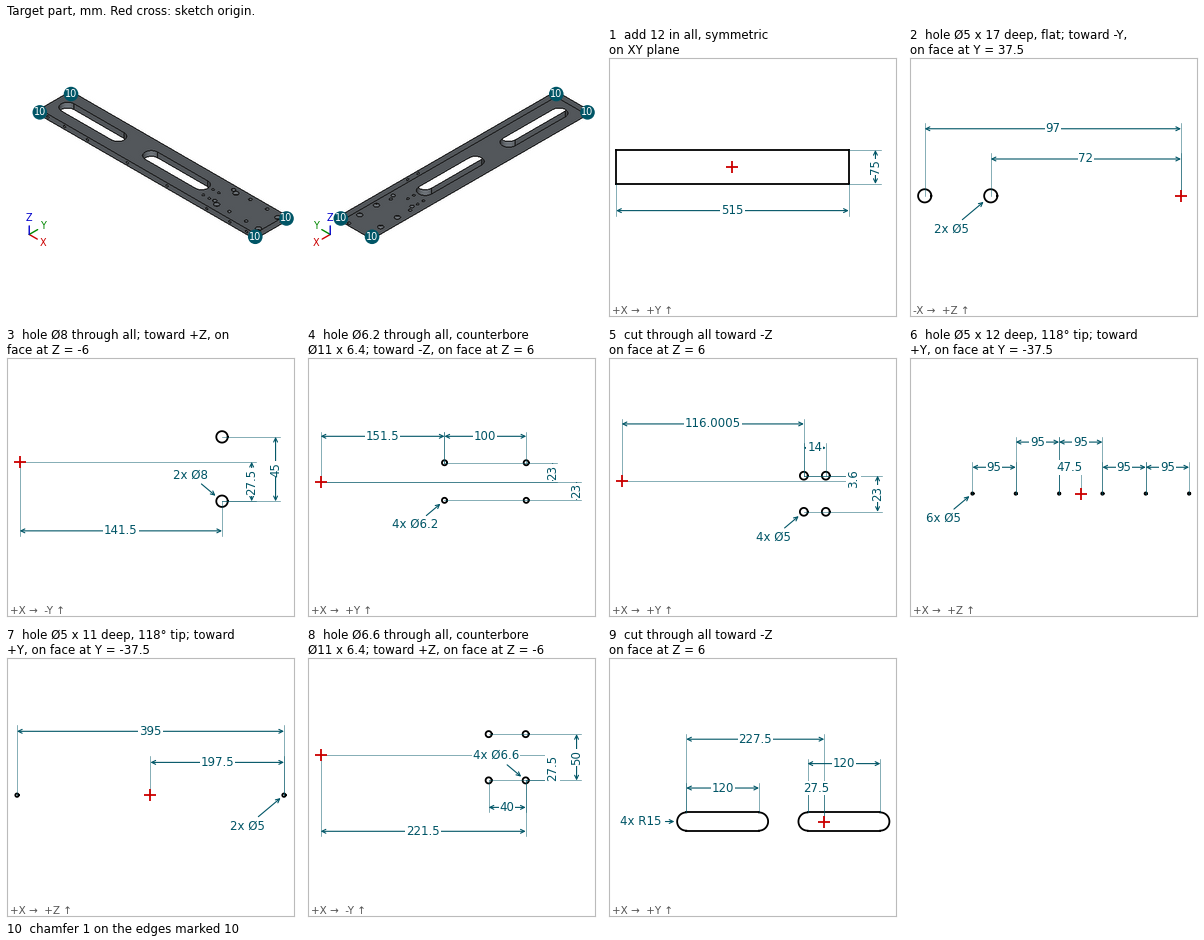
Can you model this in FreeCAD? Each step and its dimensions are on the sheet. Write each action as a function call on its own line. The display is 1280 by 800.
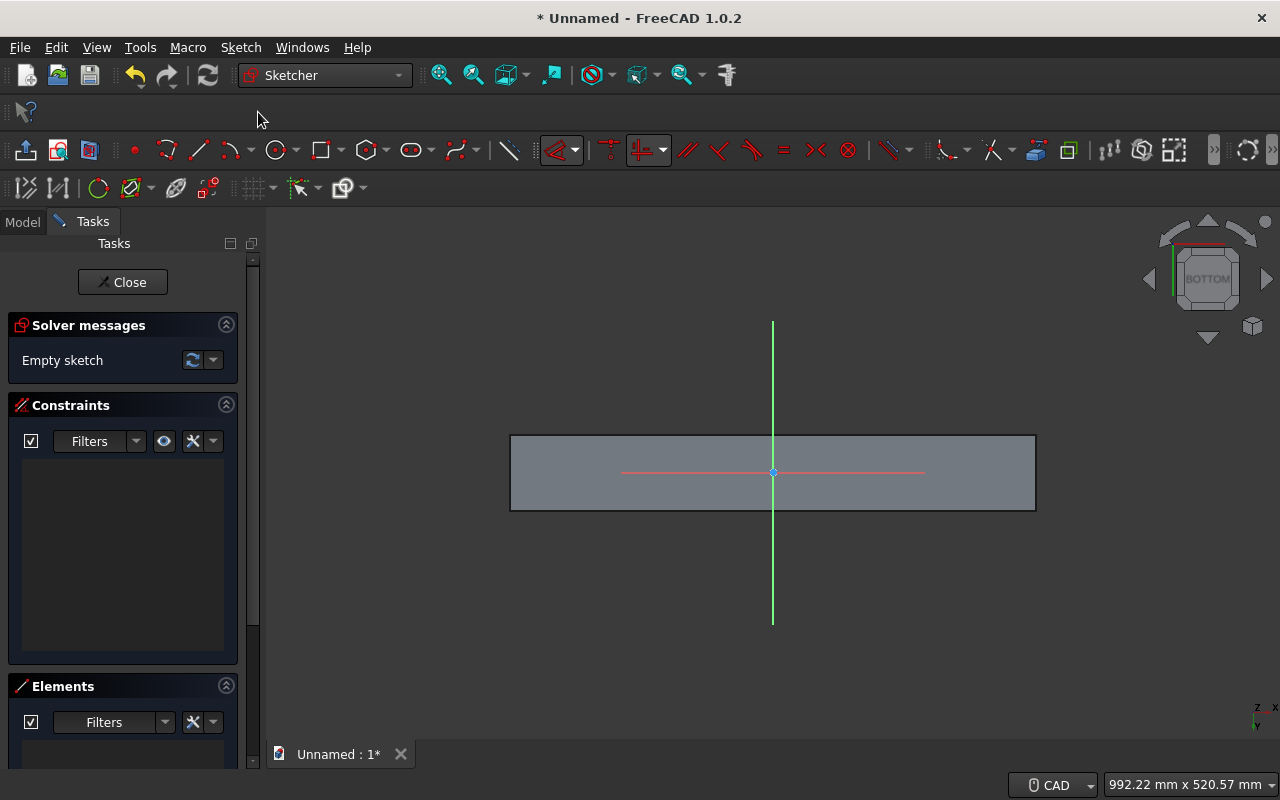
scroll(960, 479, up, 9)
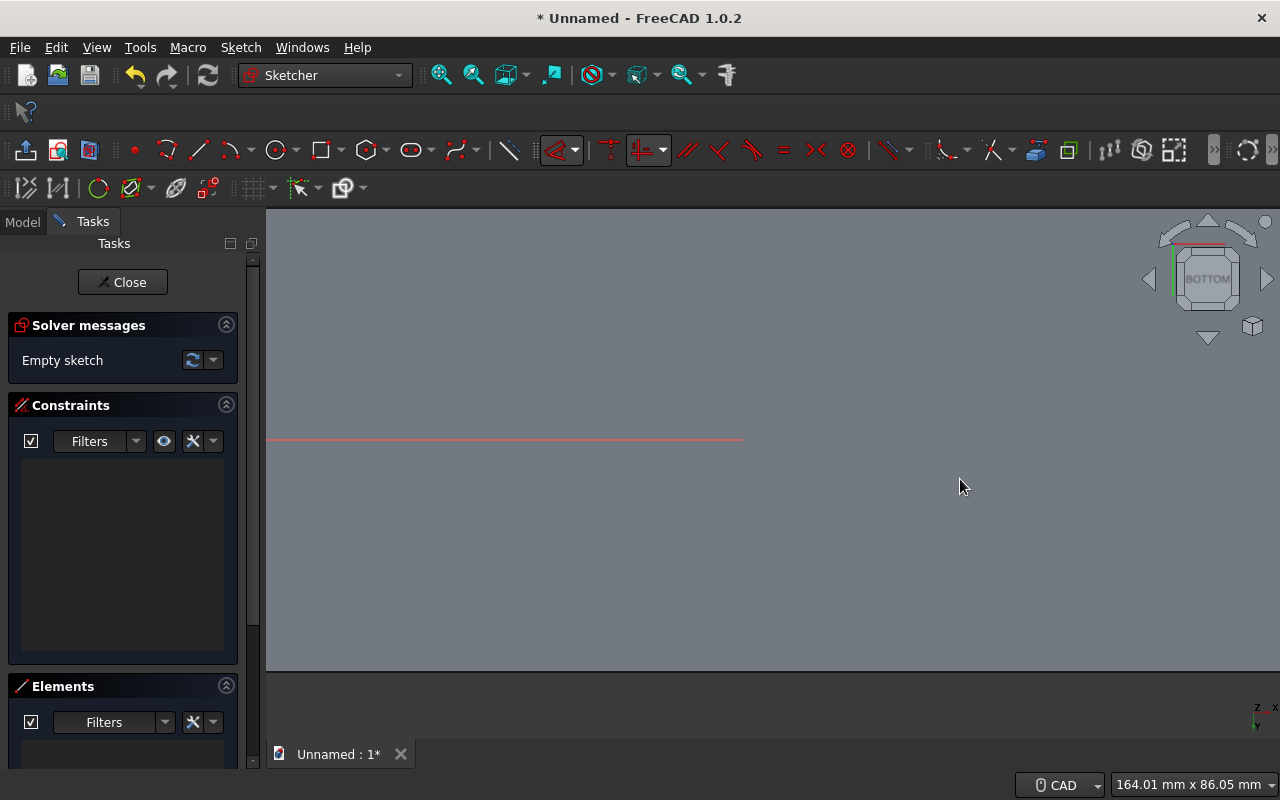
key(g)
key(c)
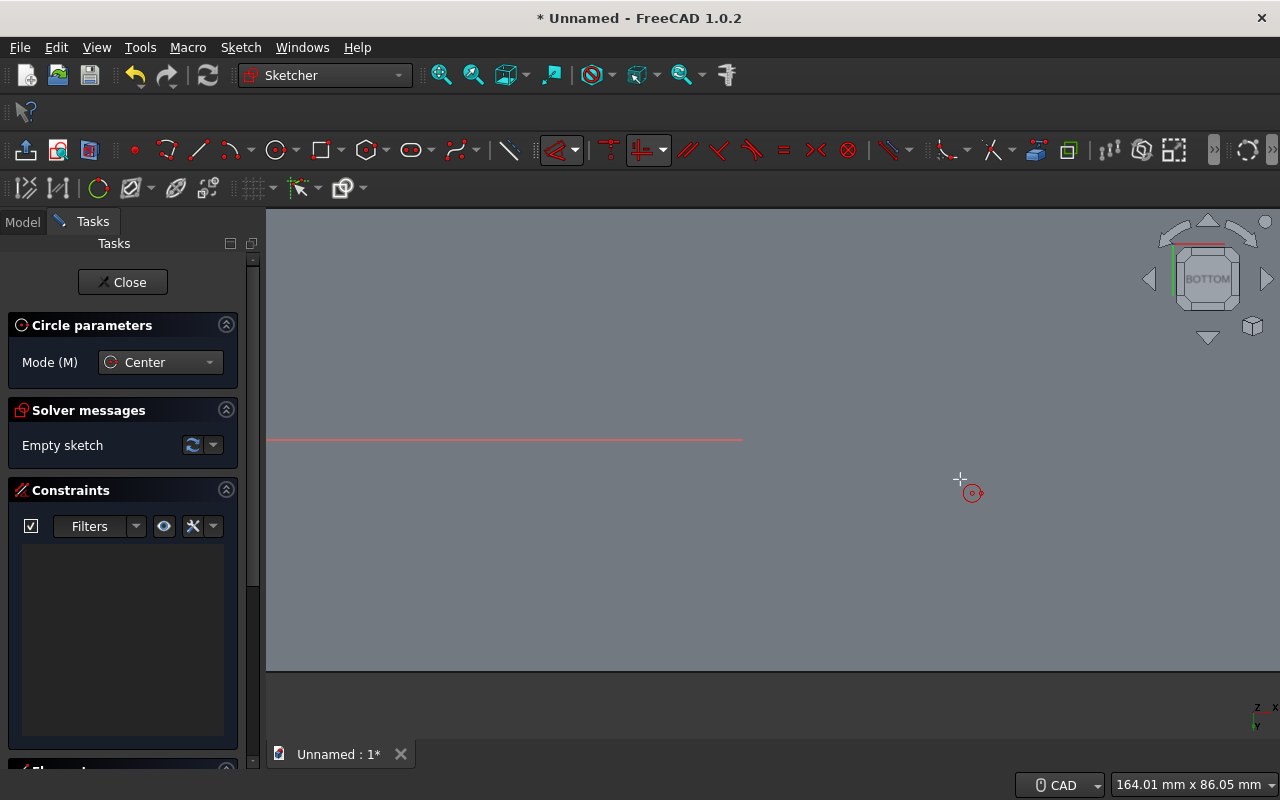
click(700, 610)
click(718, 593)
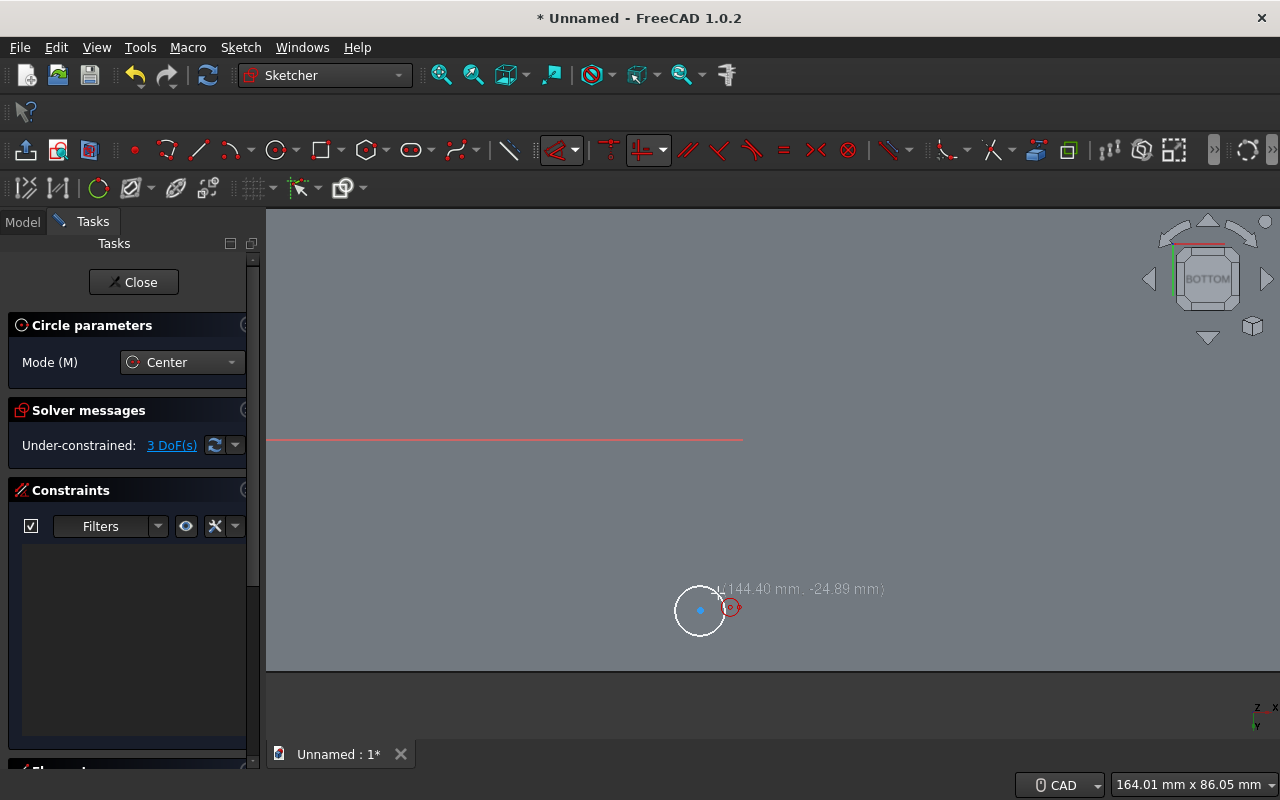
click(700, 332)
click(718, 314)
key(Escape)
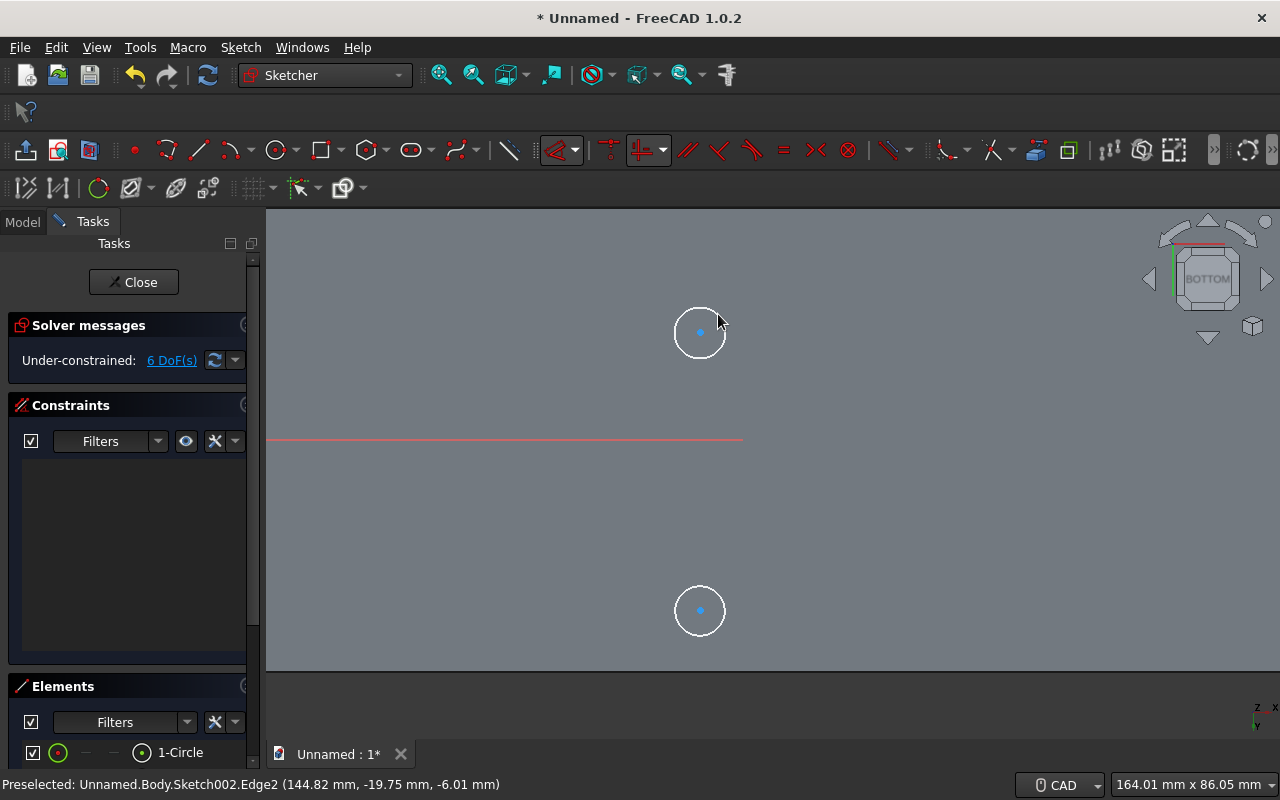
click(717, 593)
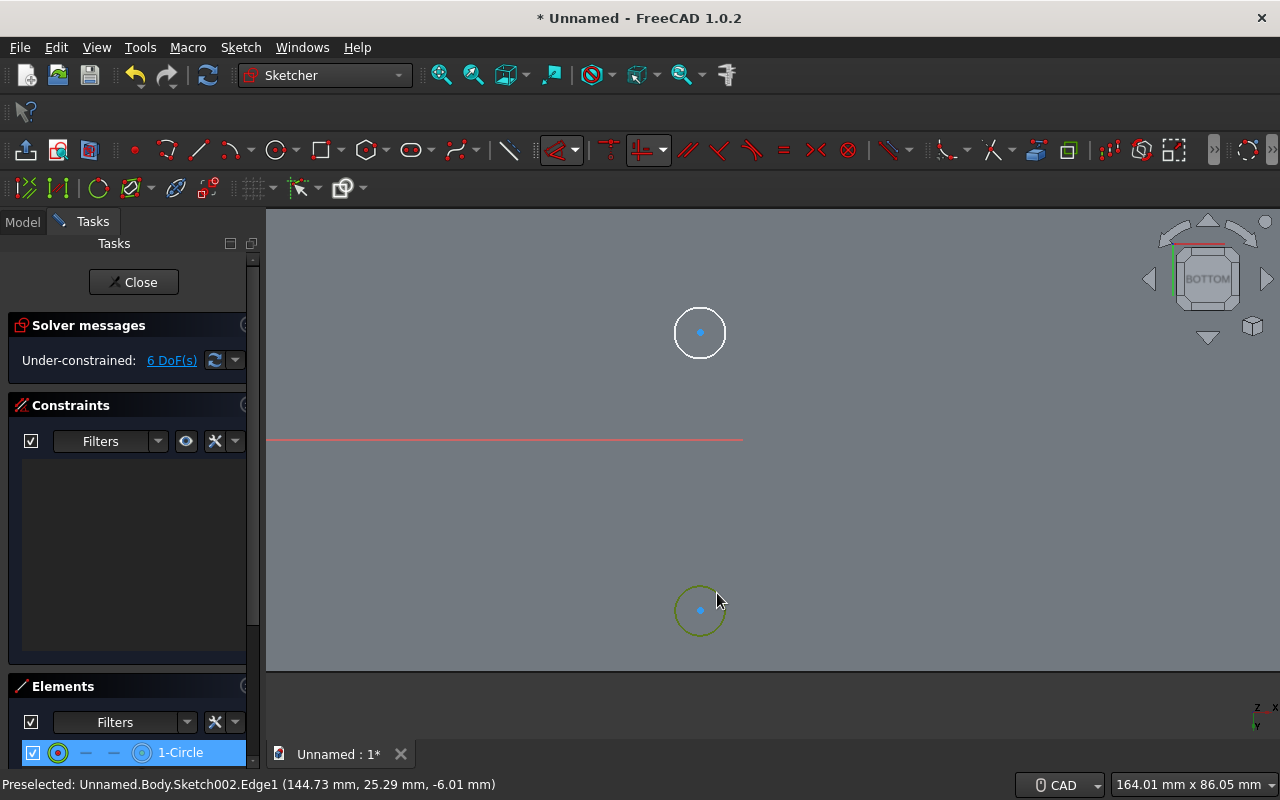
click(718, 315)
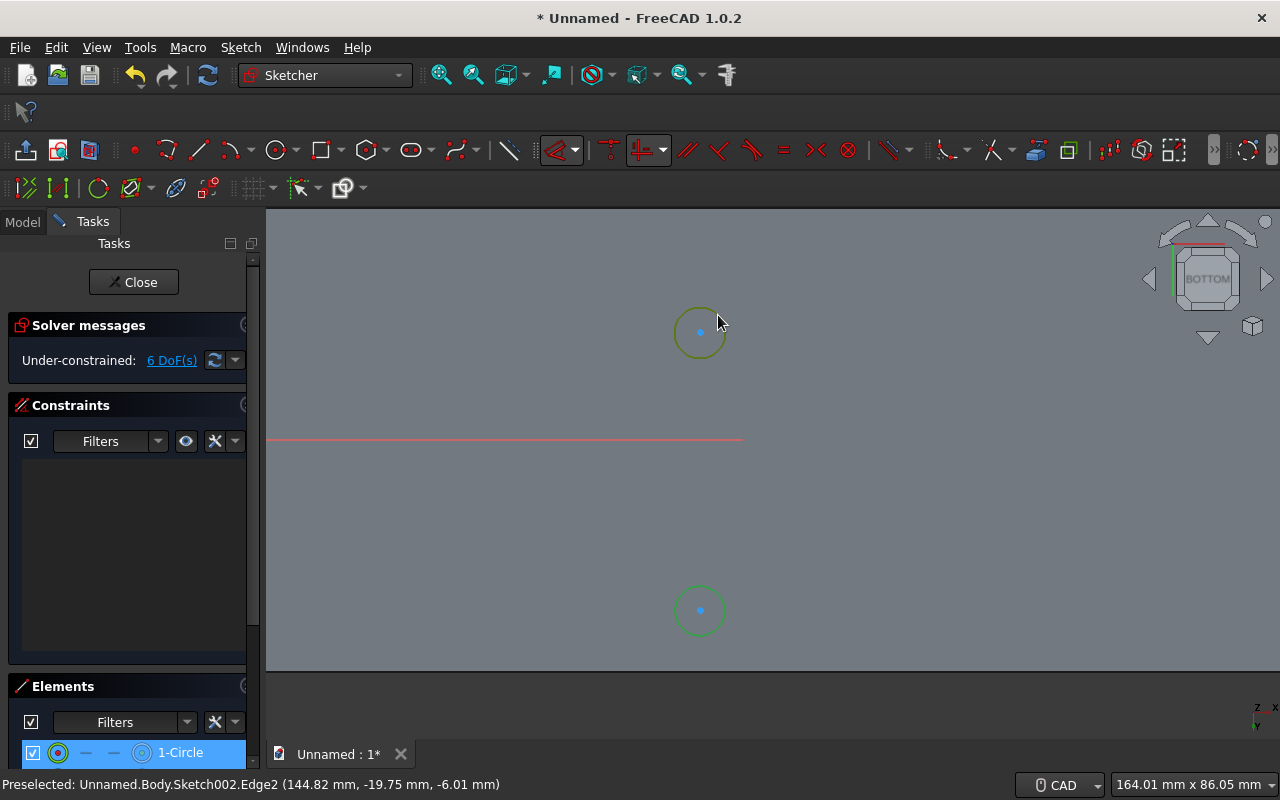
key(e)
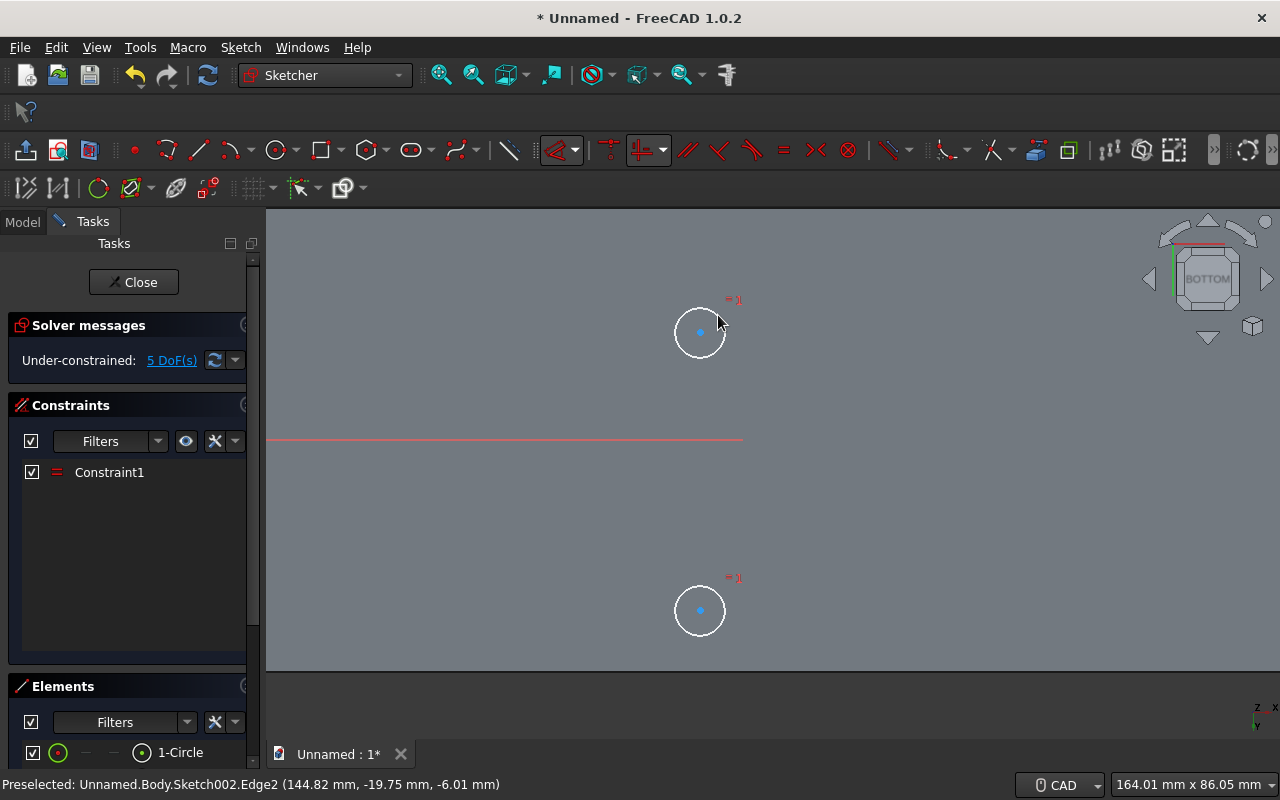
click(700, 611)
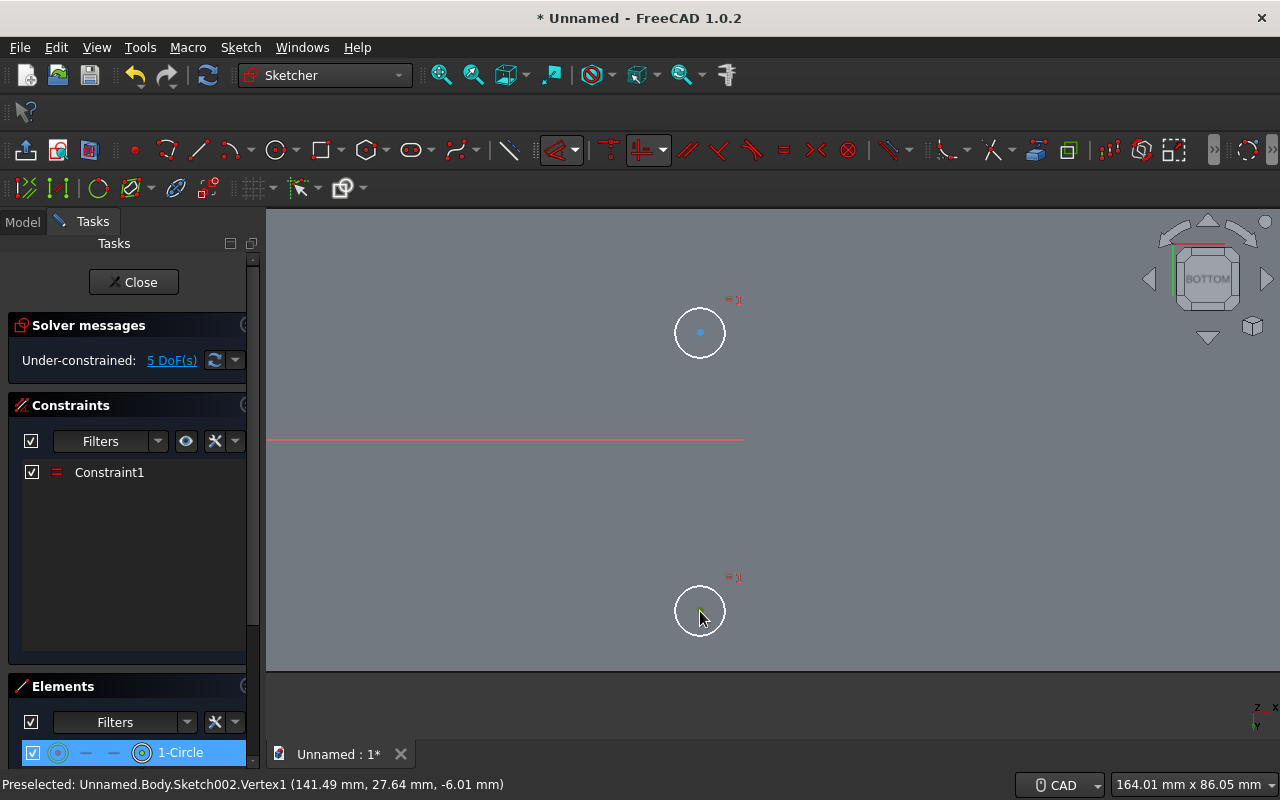
click(700, 333)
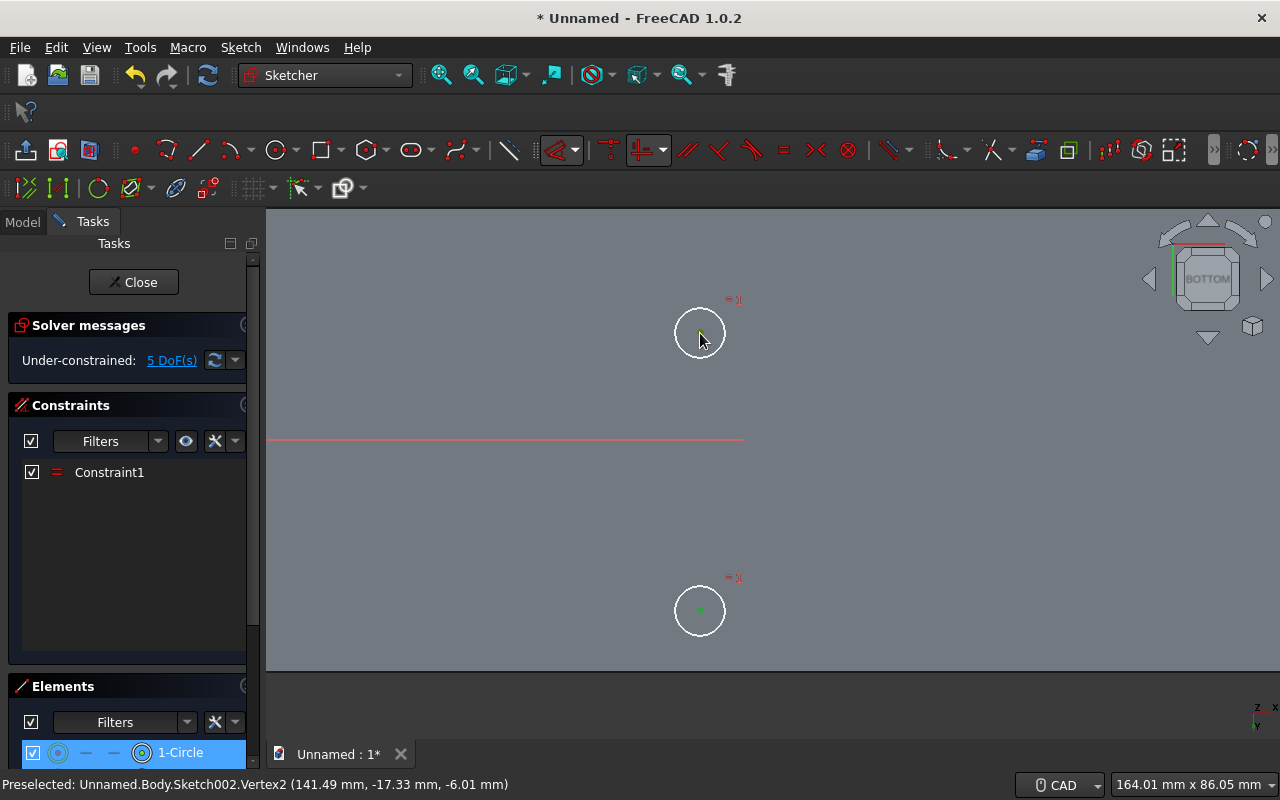
key(v)